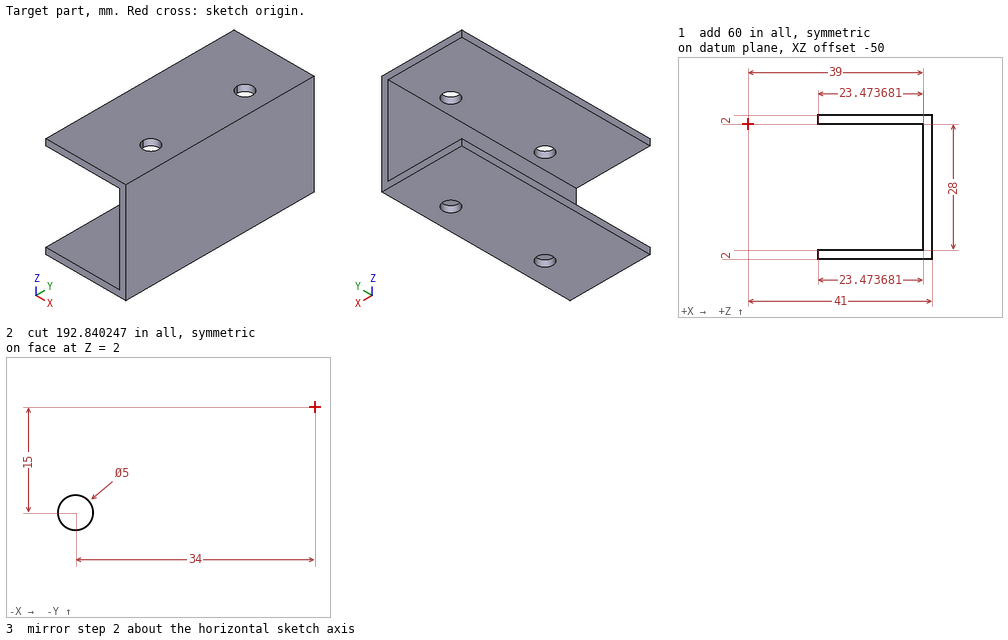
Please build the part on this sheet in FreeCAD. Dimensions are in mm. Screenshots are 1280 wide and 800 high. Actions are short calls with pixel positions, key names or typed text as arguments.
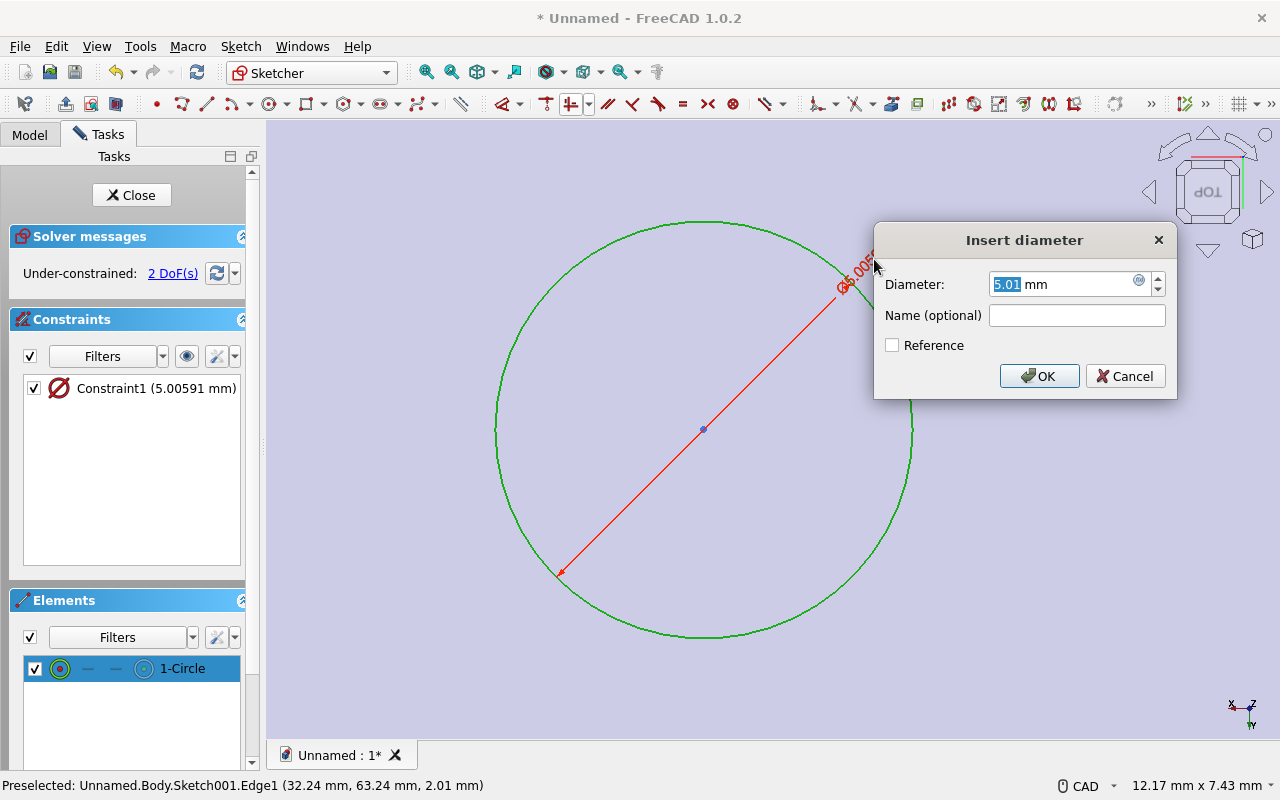
text(5)
key(Return)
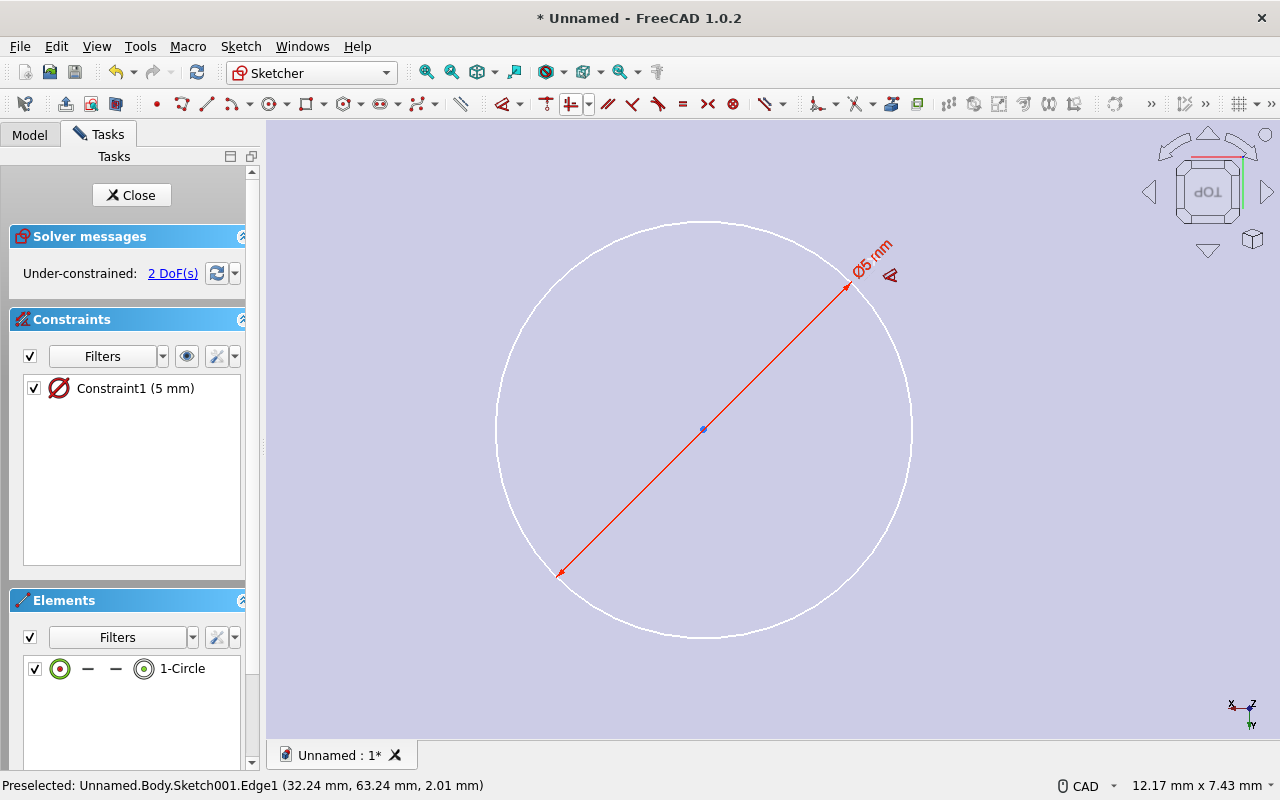
click(704, 430)
click(815, 464)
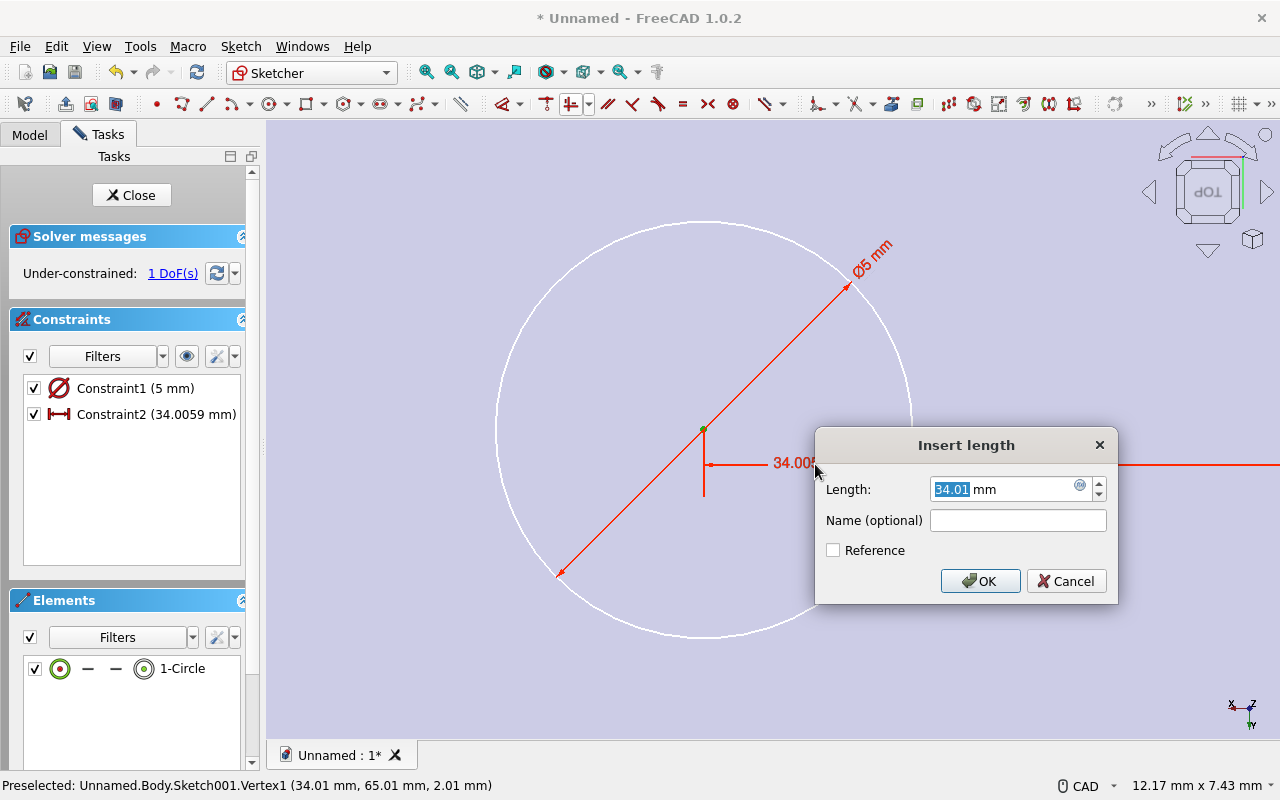
text(34)
key(Return)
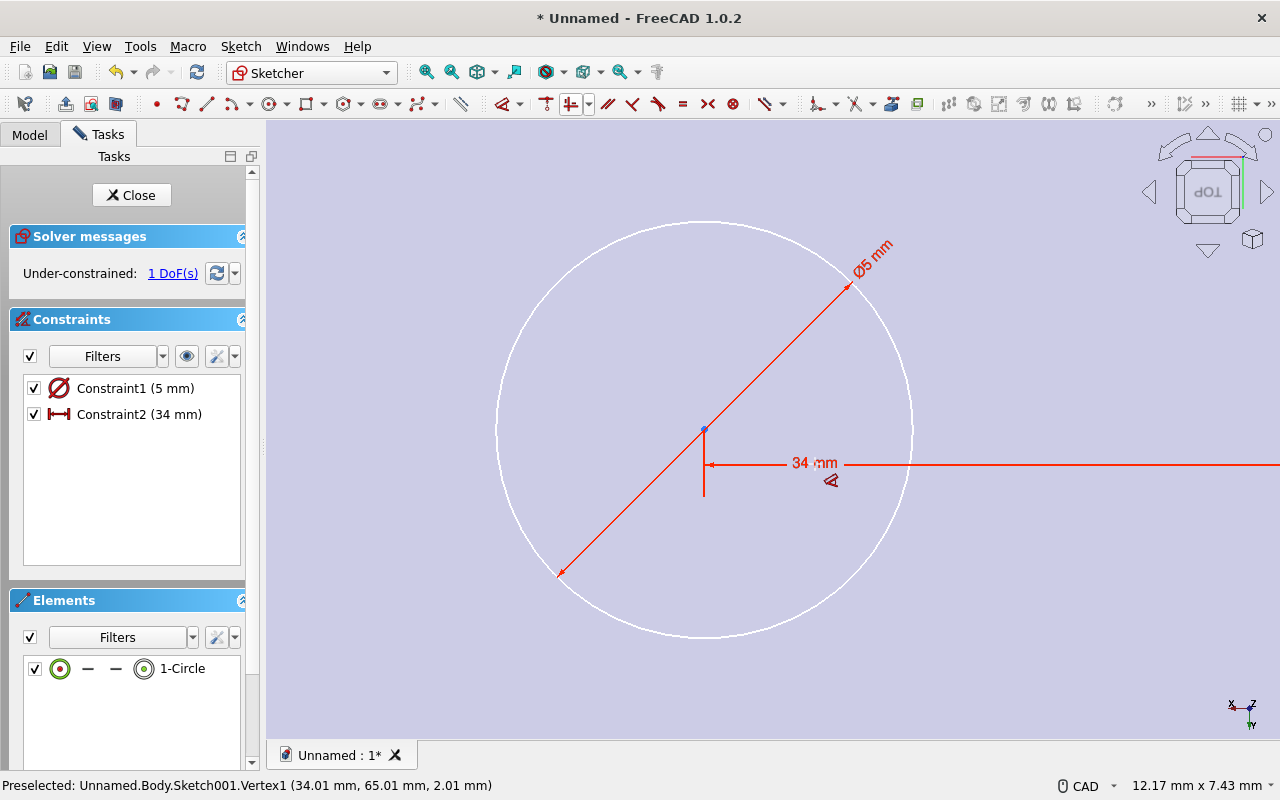
click(704, 430)
click(670, 289)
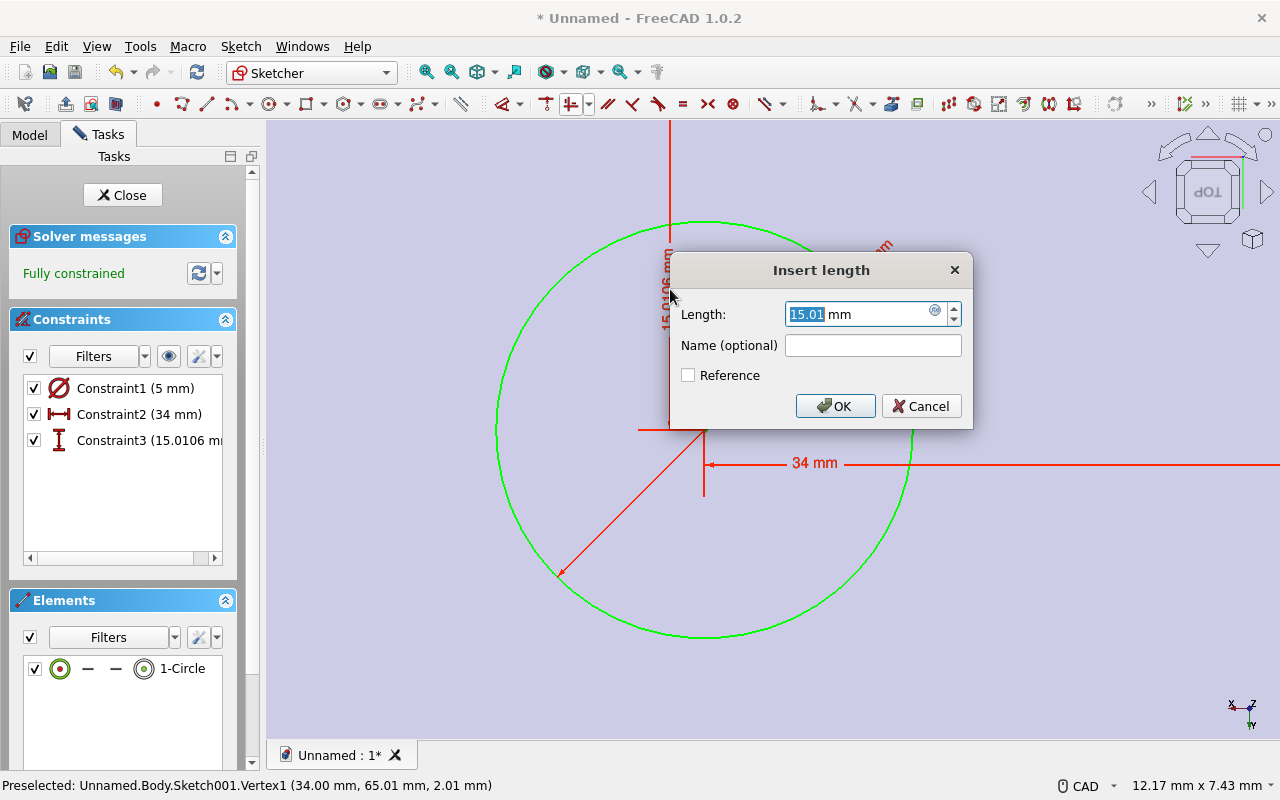
text(15)
key(Return)
key(Escape)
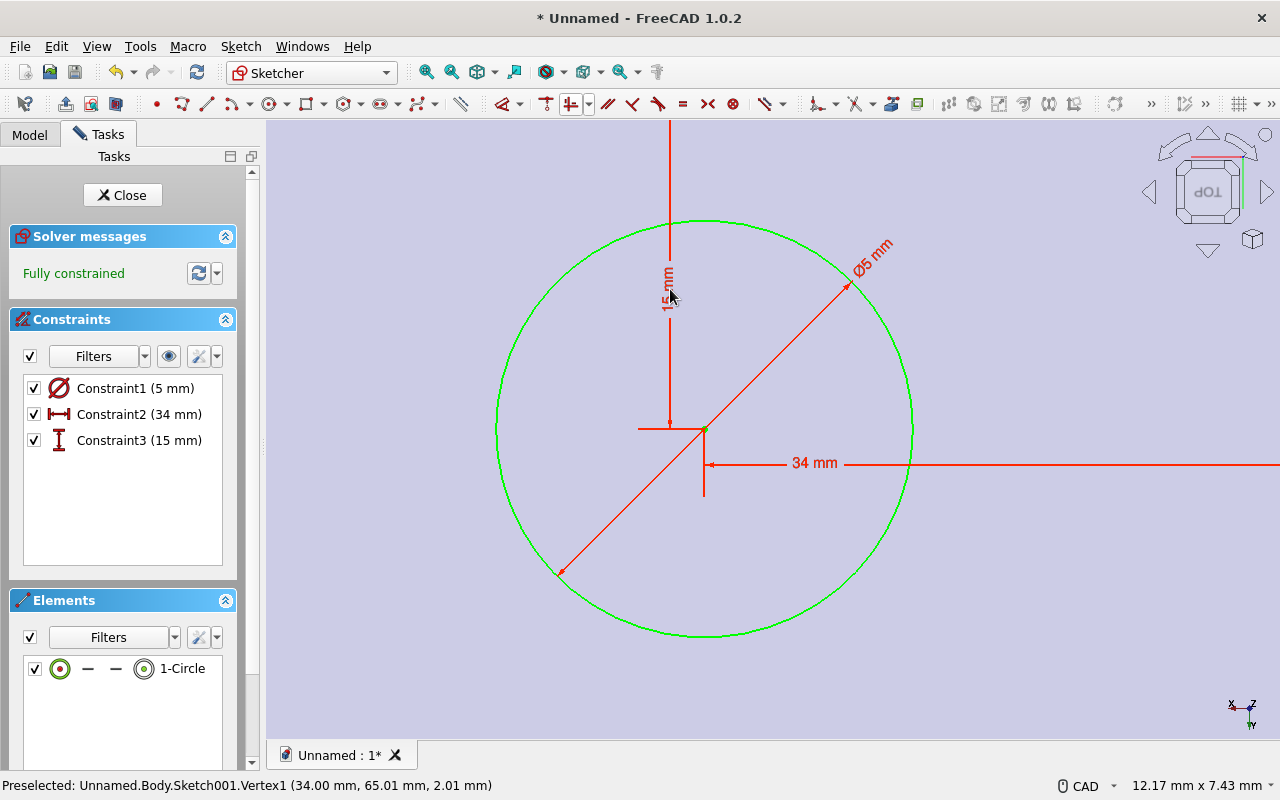
click(123, 195)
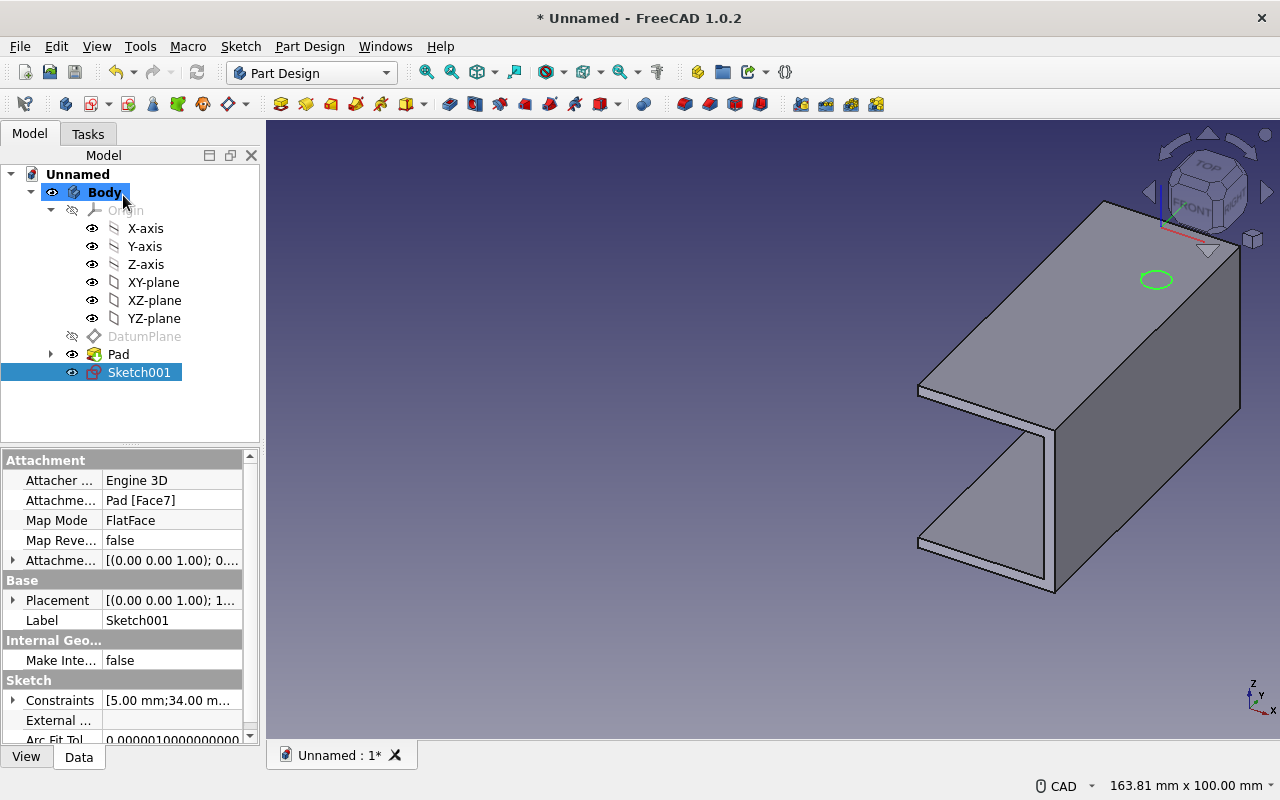
click(450, 104)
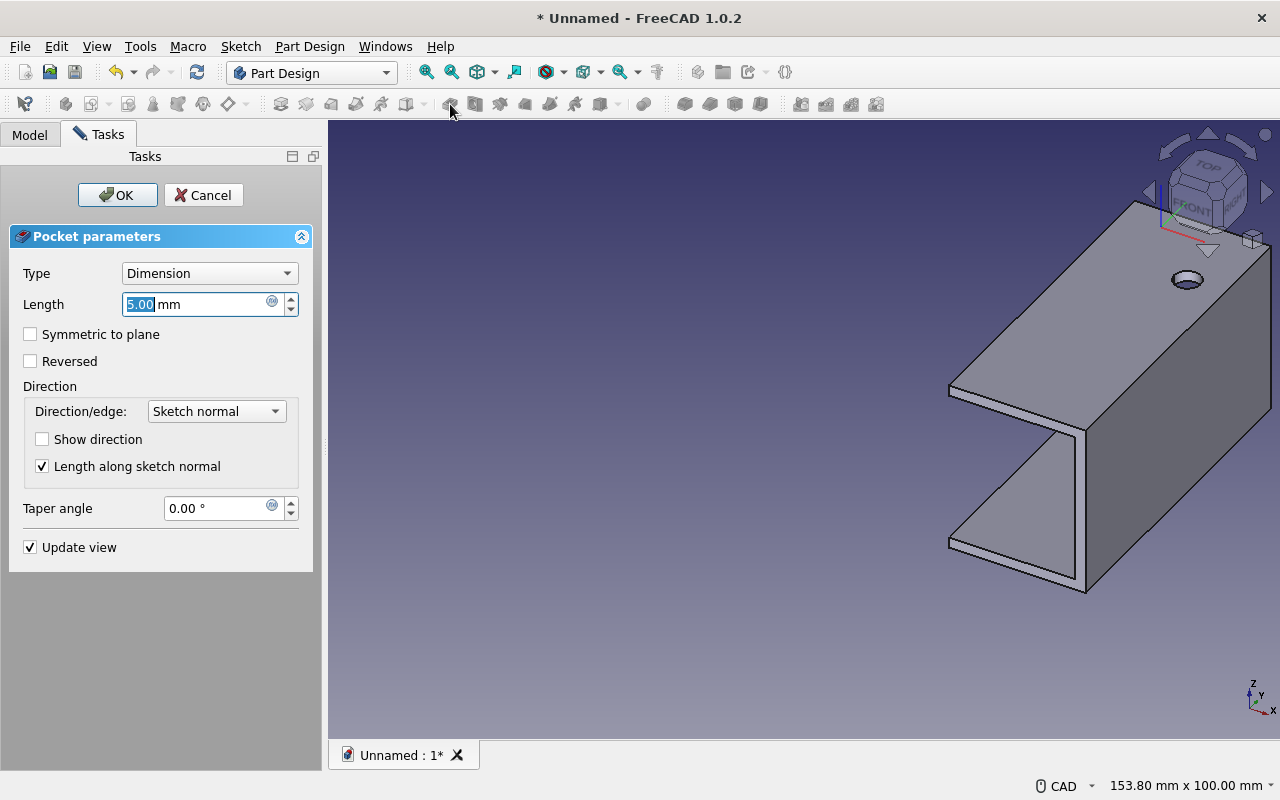
text(192.840247)
key(Tab)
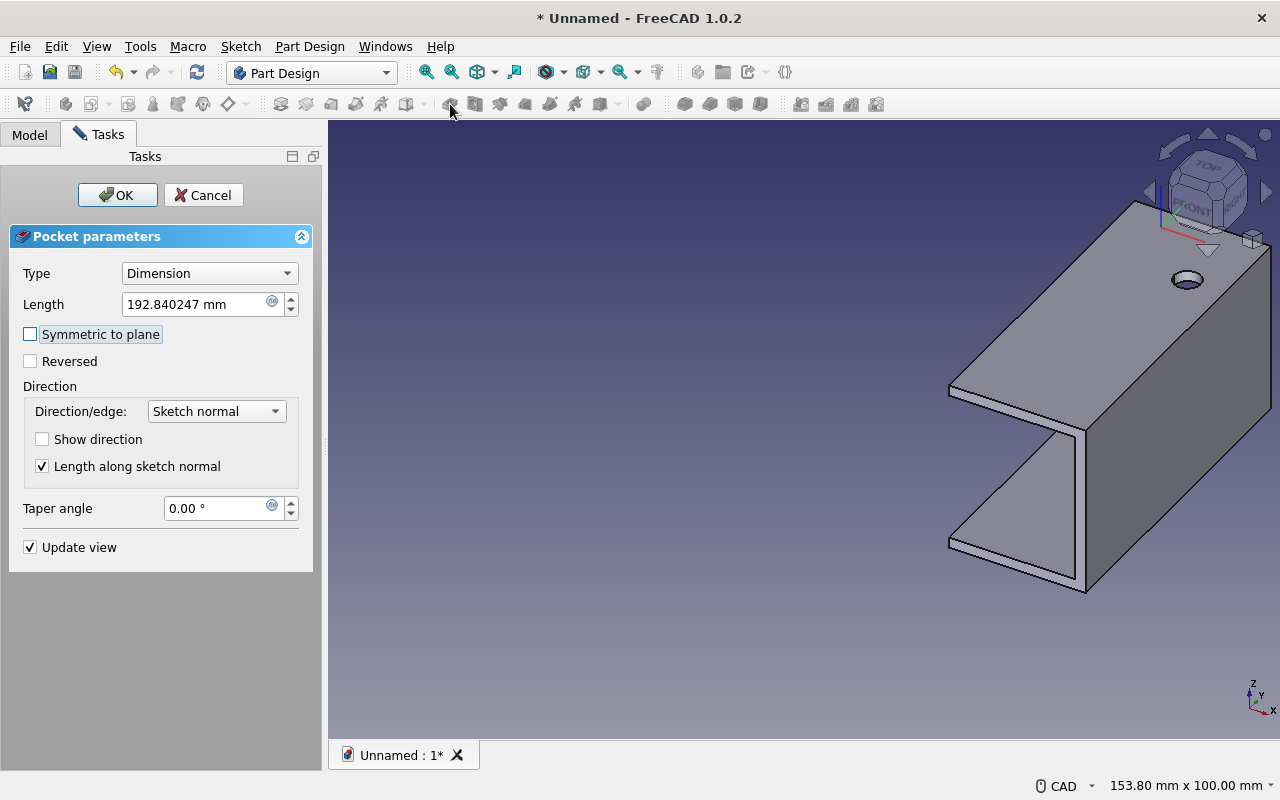
click(31, 334)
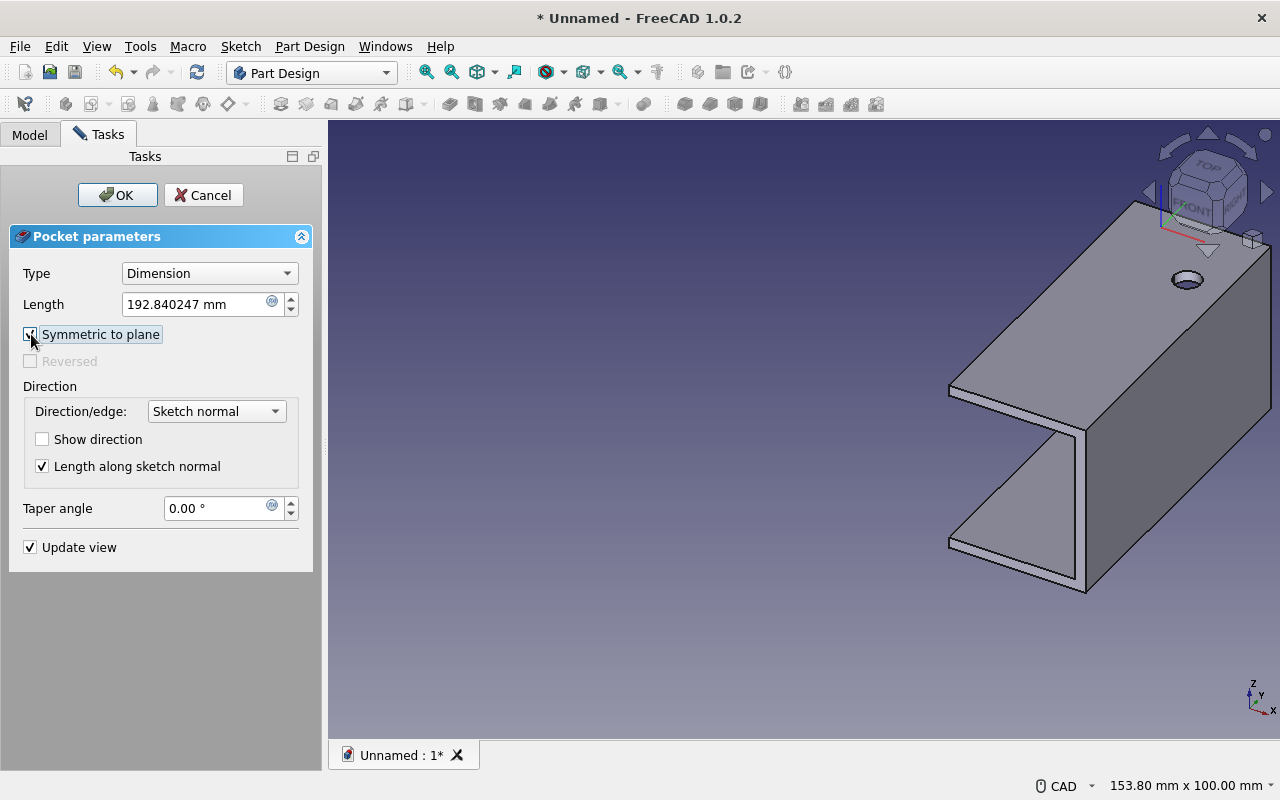
click(118, 195)